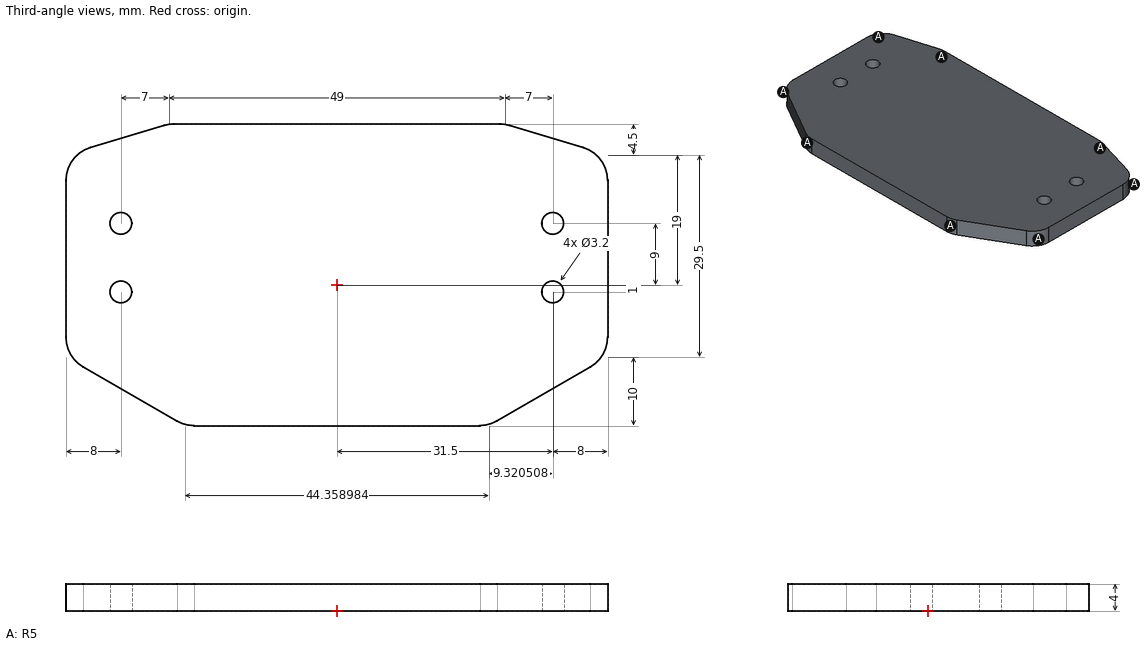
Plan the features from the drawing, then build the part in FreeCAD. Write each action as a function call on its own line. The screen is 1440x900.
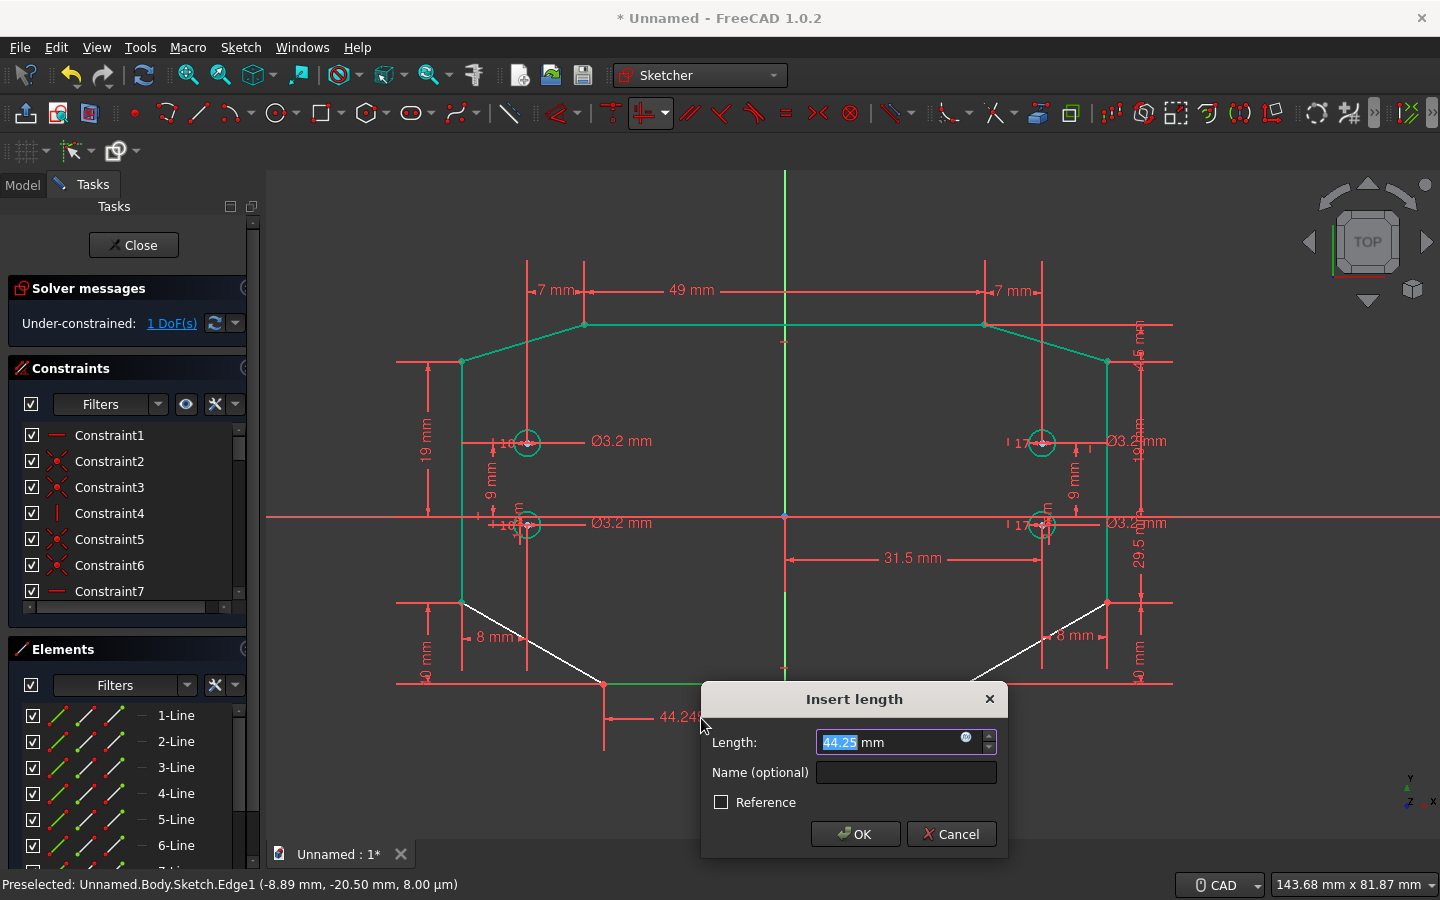
text(44.358984)
key(Return)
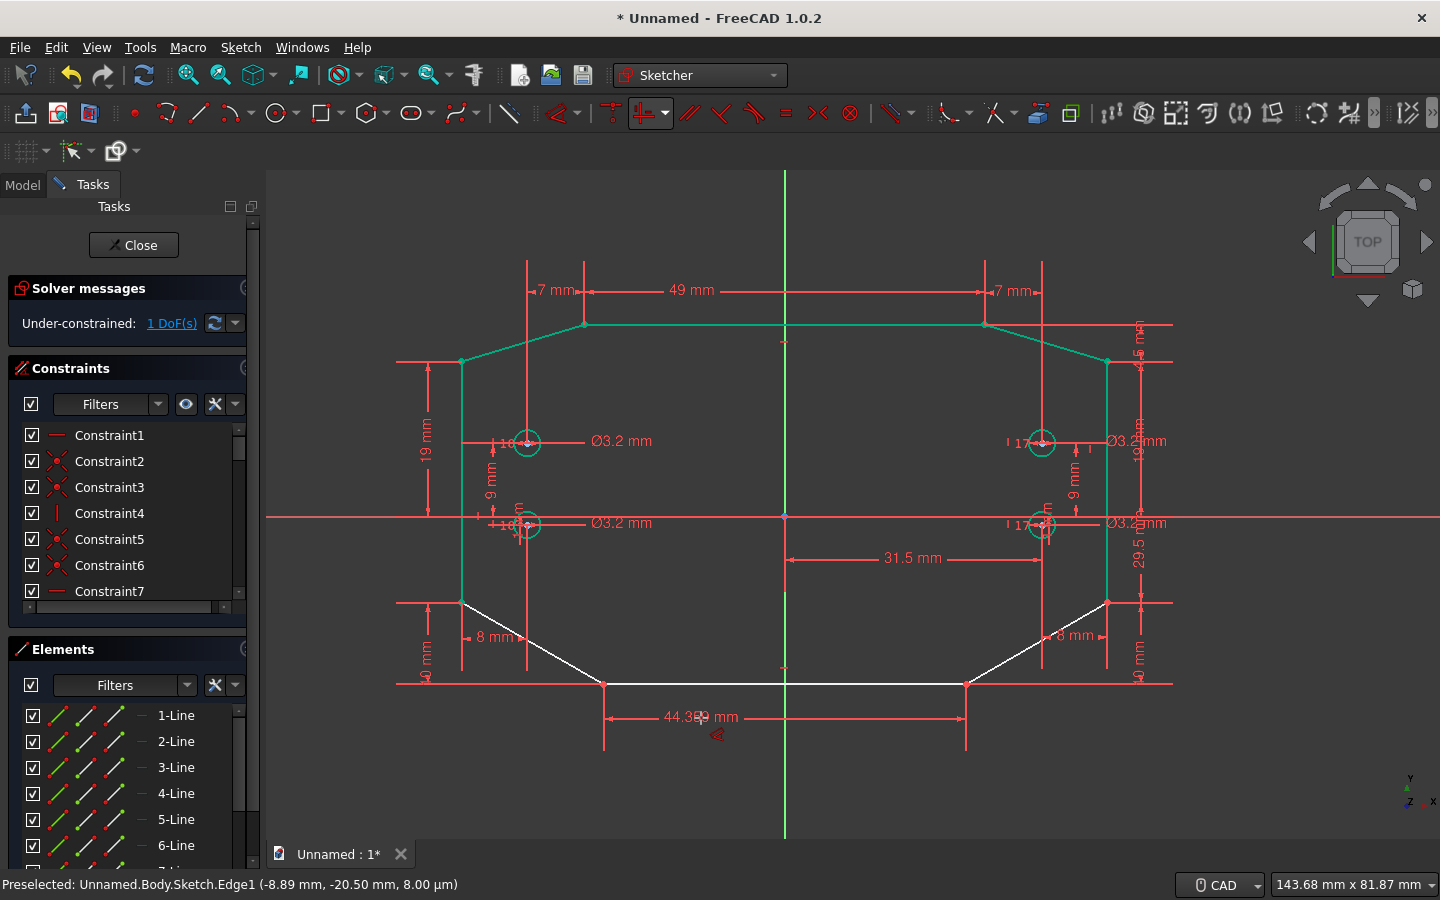
click(966, 684)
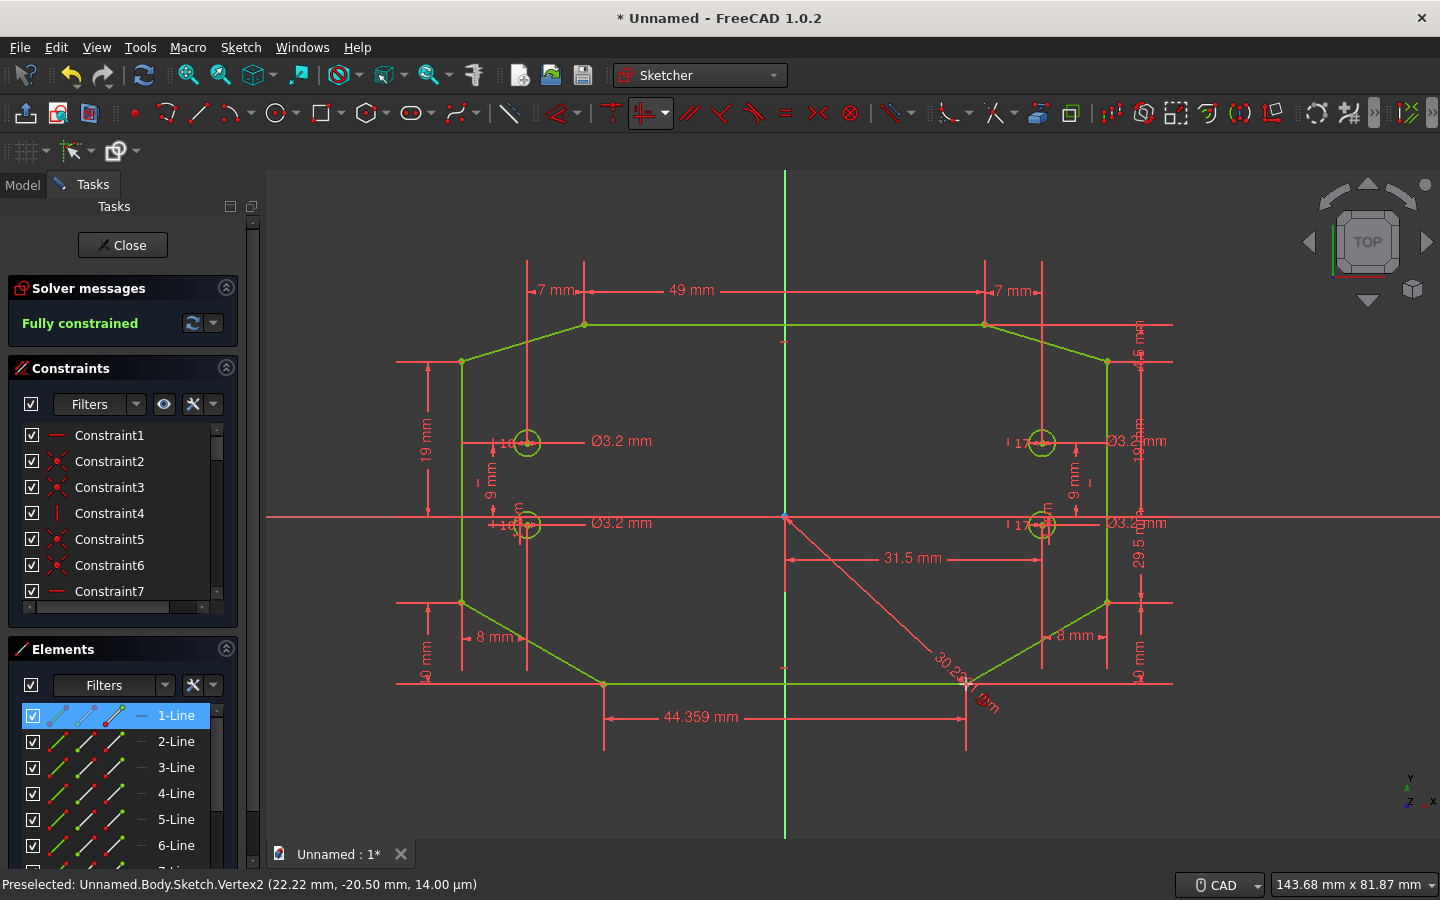
click(1042, 525)
click(1004, 718)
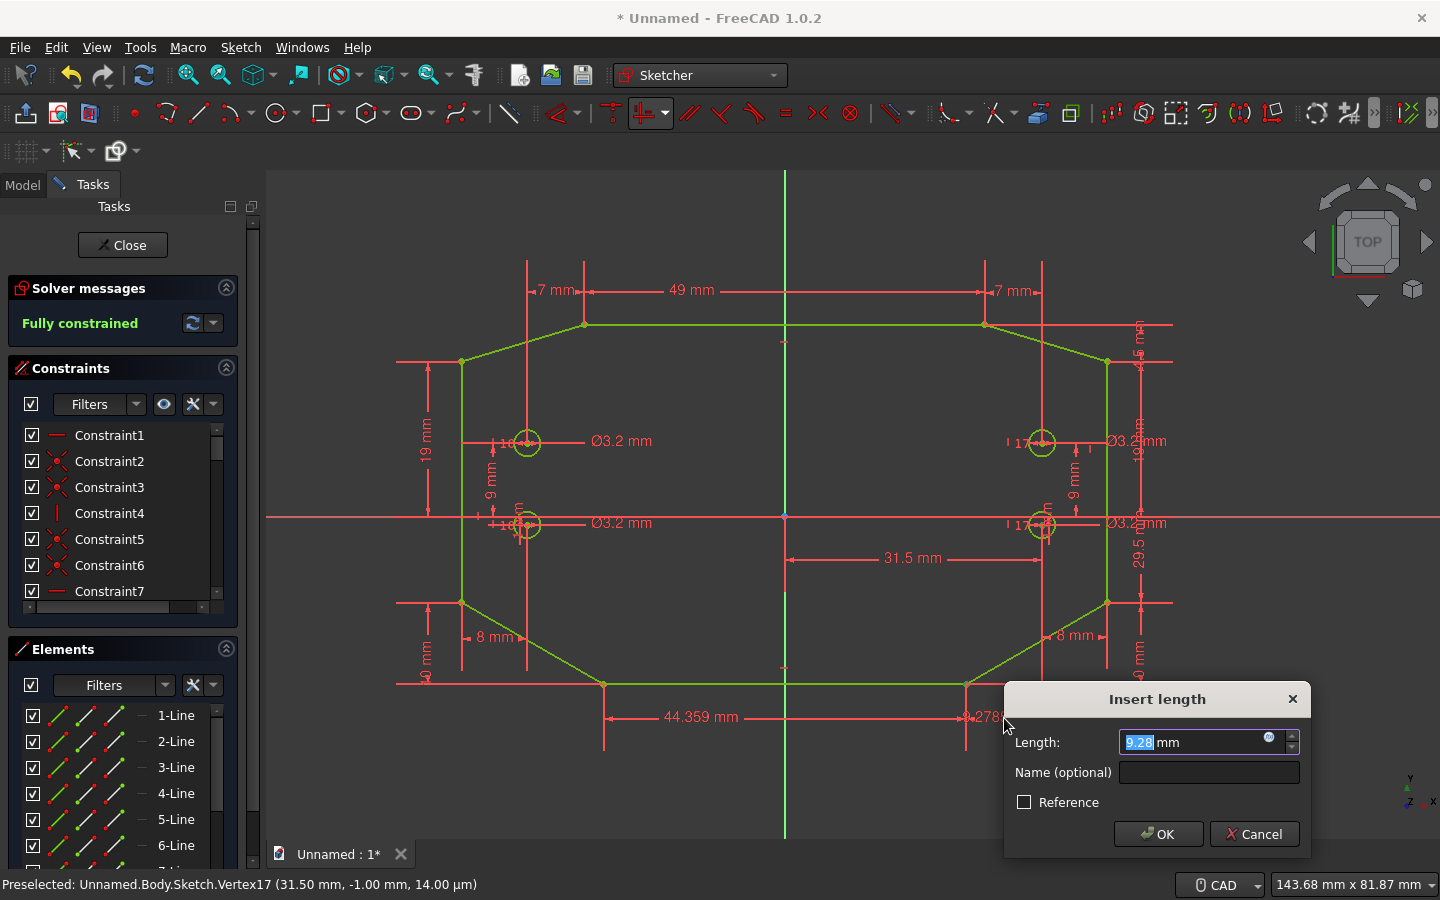
text(9.320508)
key(Return)
key(Escape)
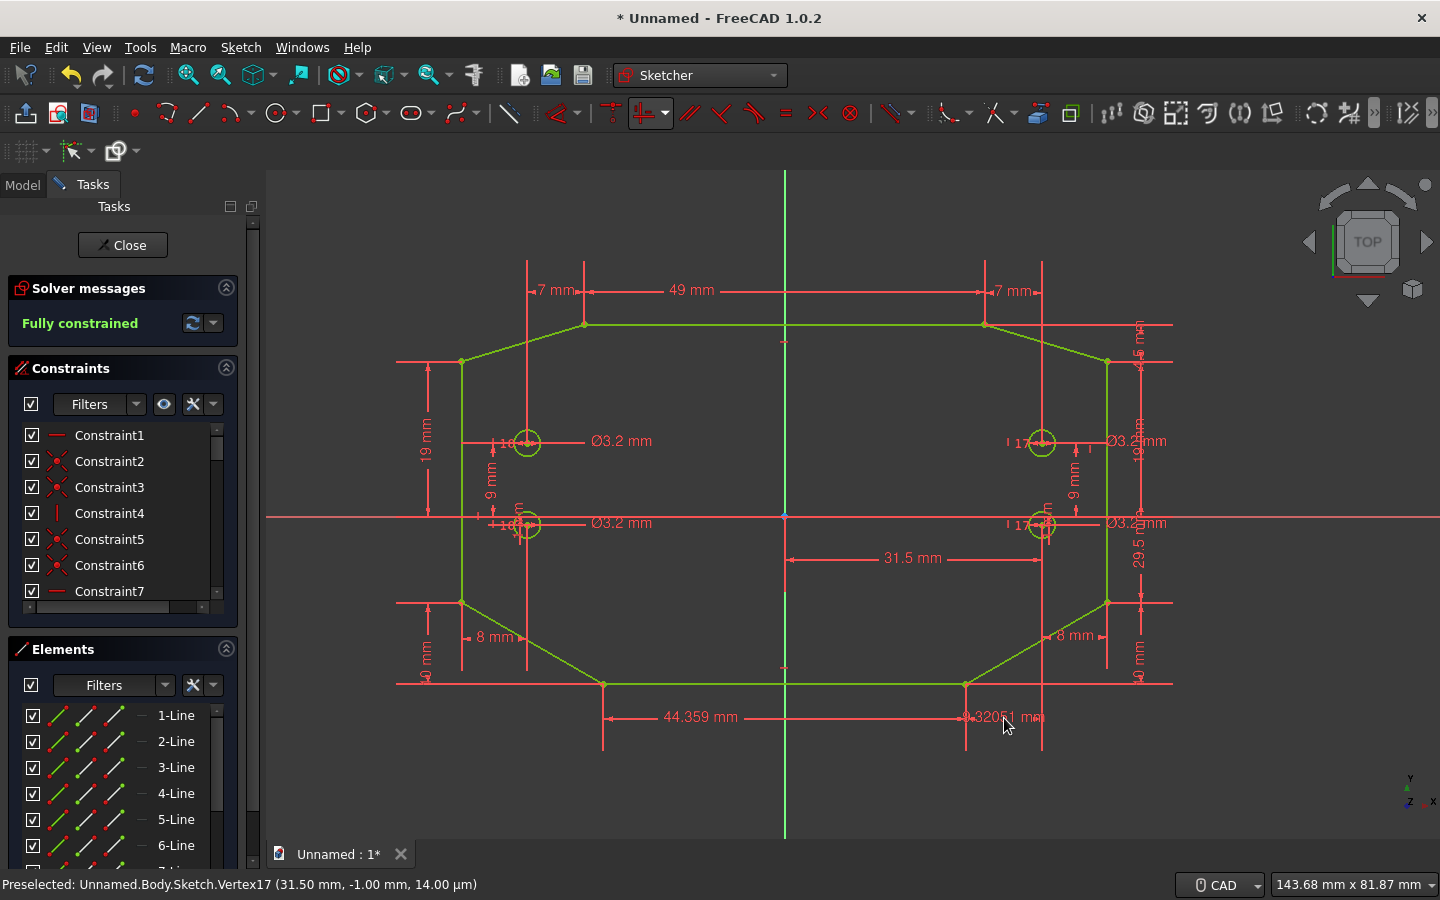
click(123, 245)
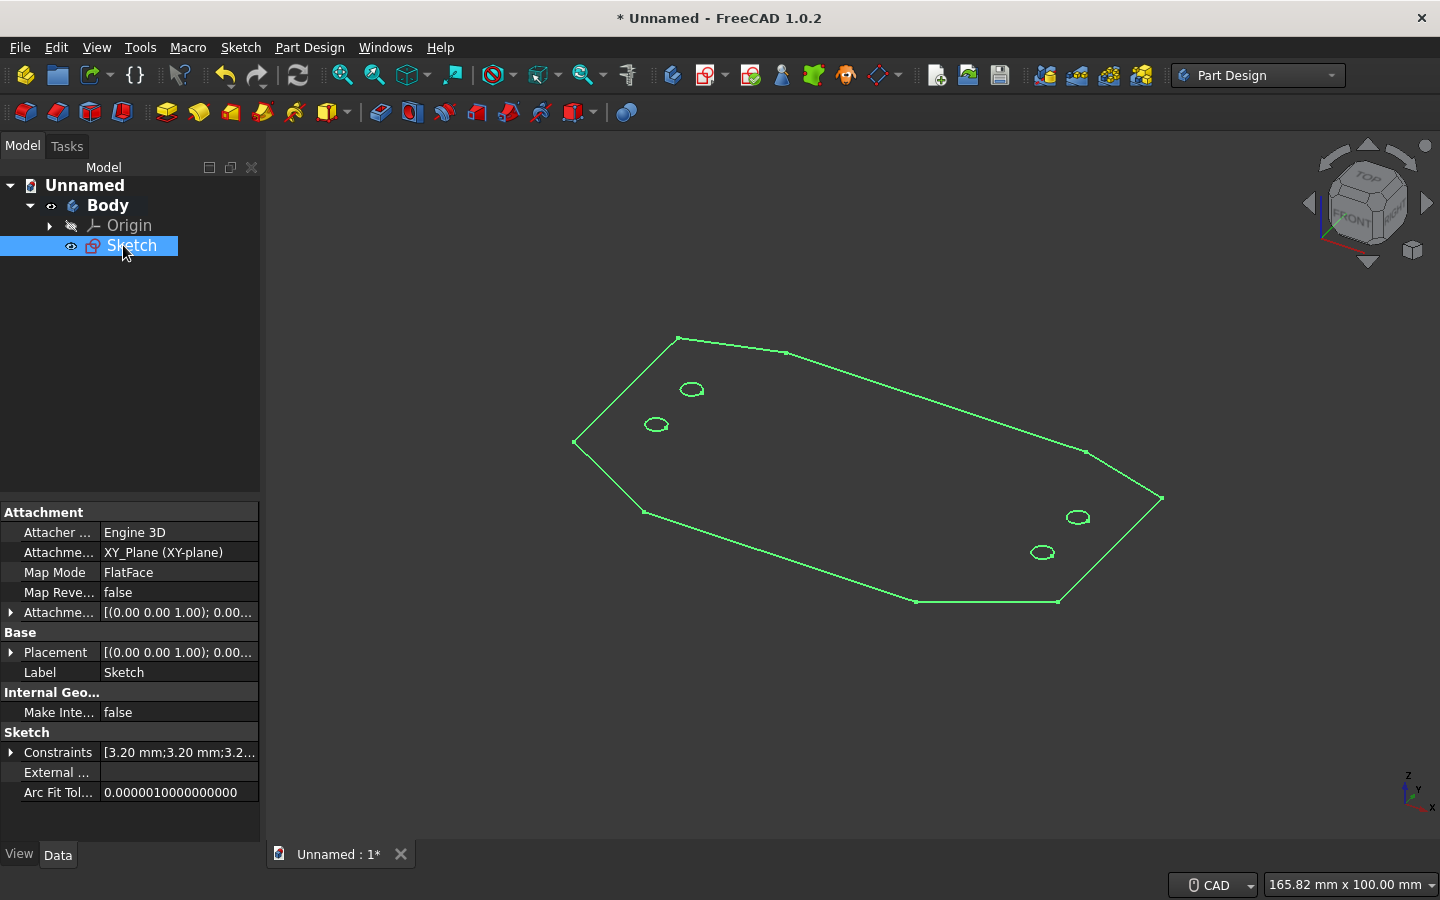
click(168, 112)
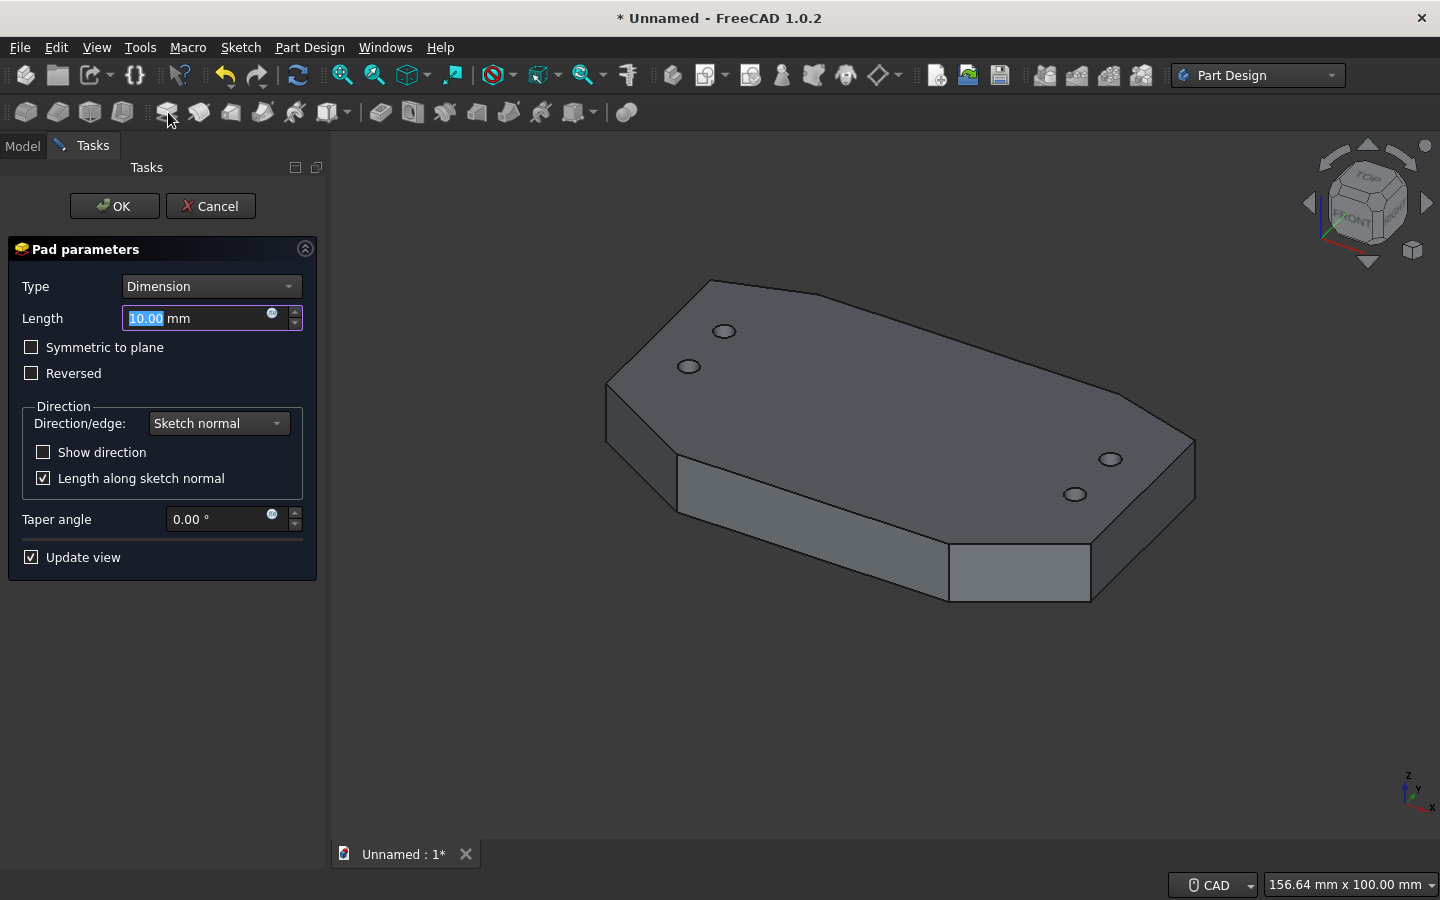
text(4)
key(Tab)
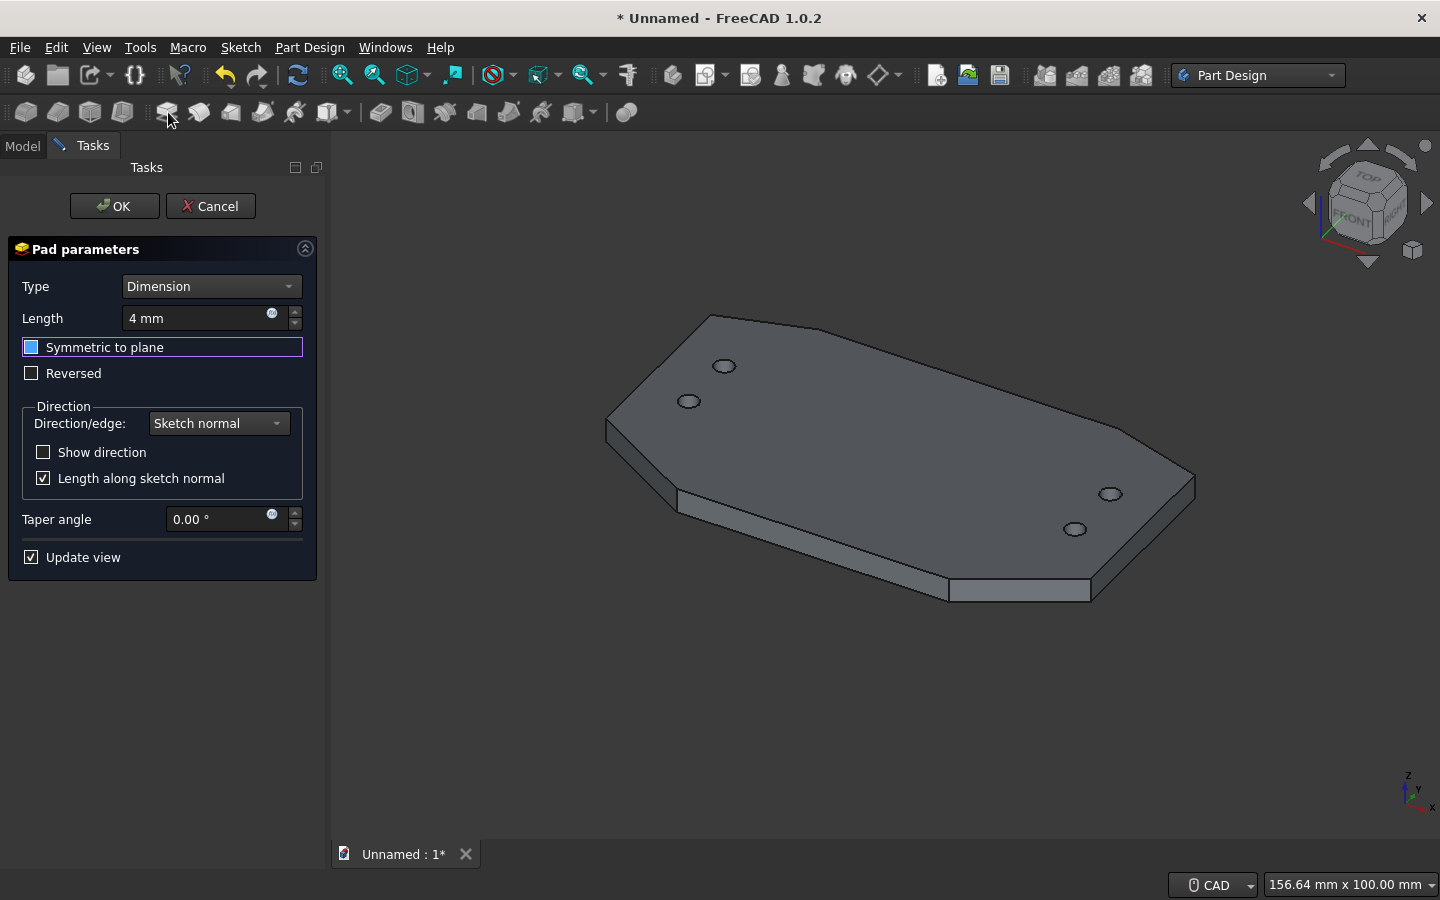
click(115, 206)